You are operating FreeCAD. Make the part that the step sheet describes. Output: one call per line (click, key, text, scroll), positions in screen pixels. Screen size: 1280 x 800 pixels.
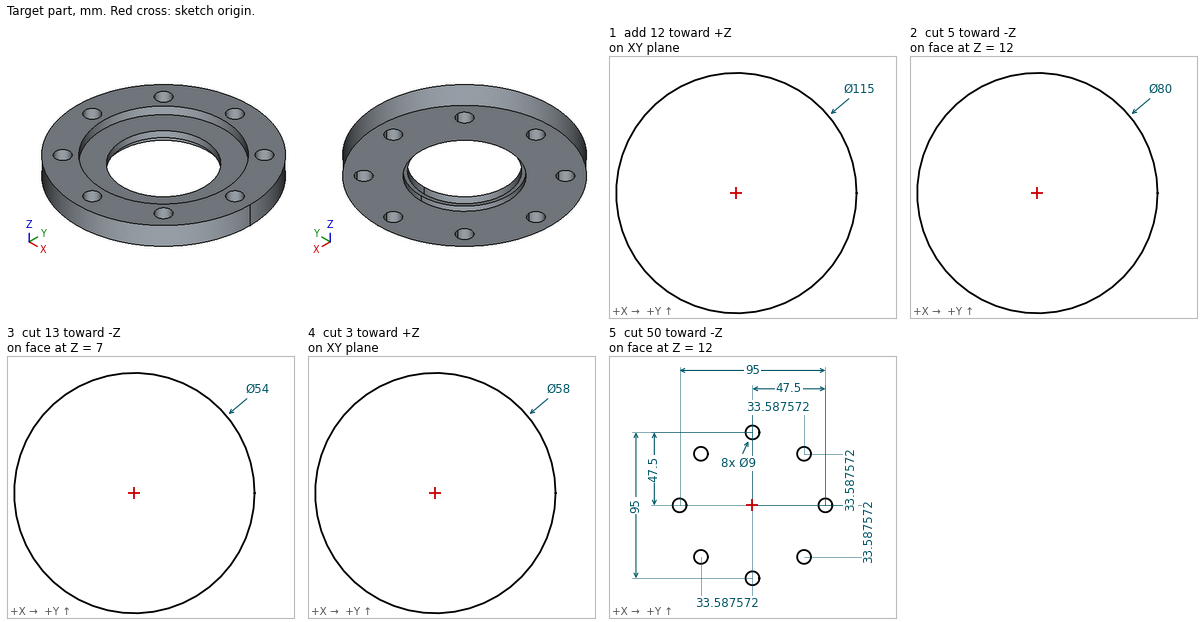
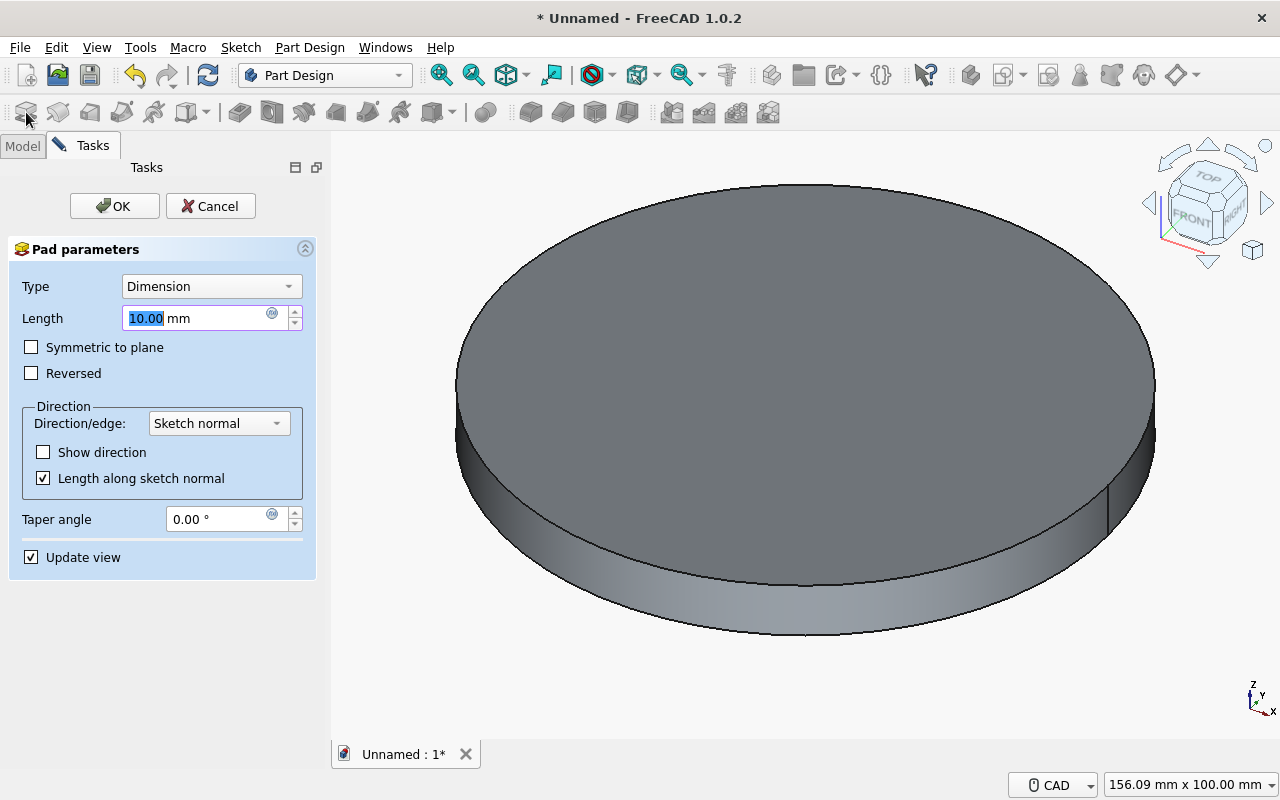
text(12)
key(Tab)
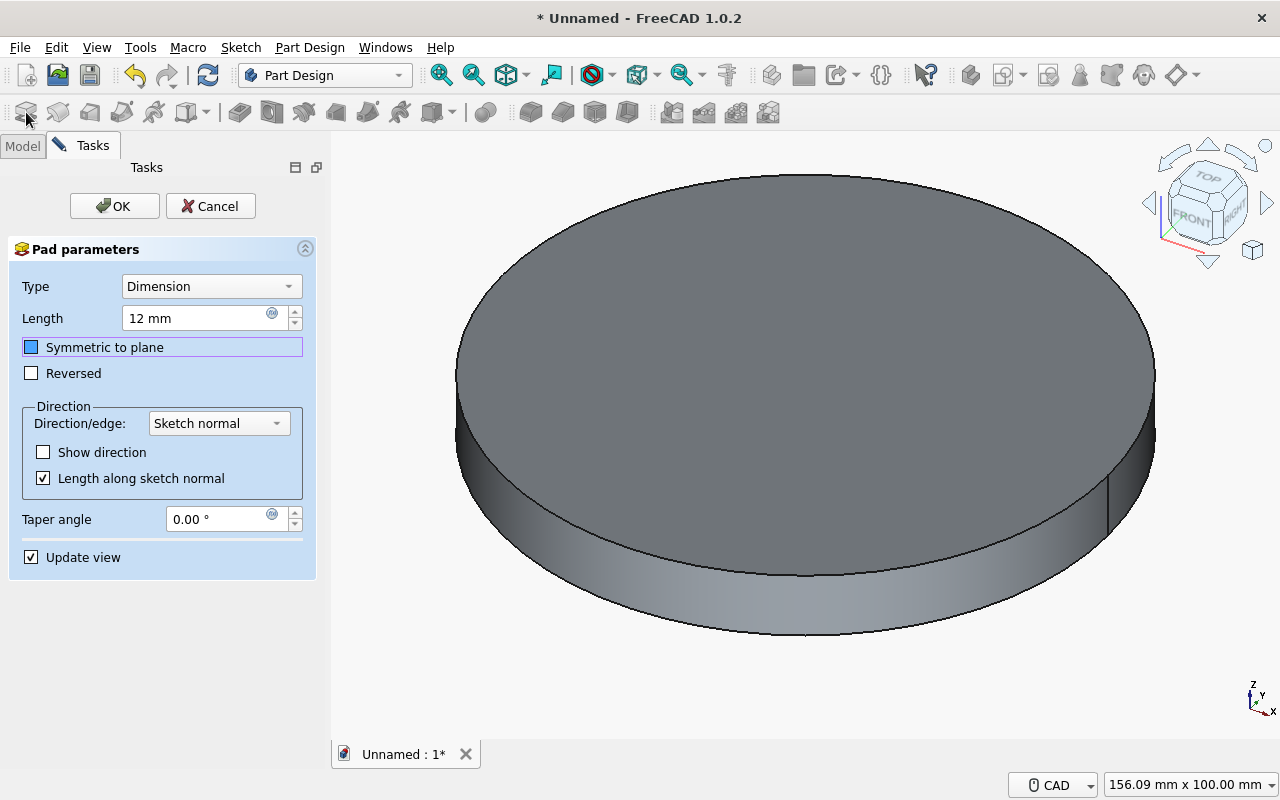
click(115, 206)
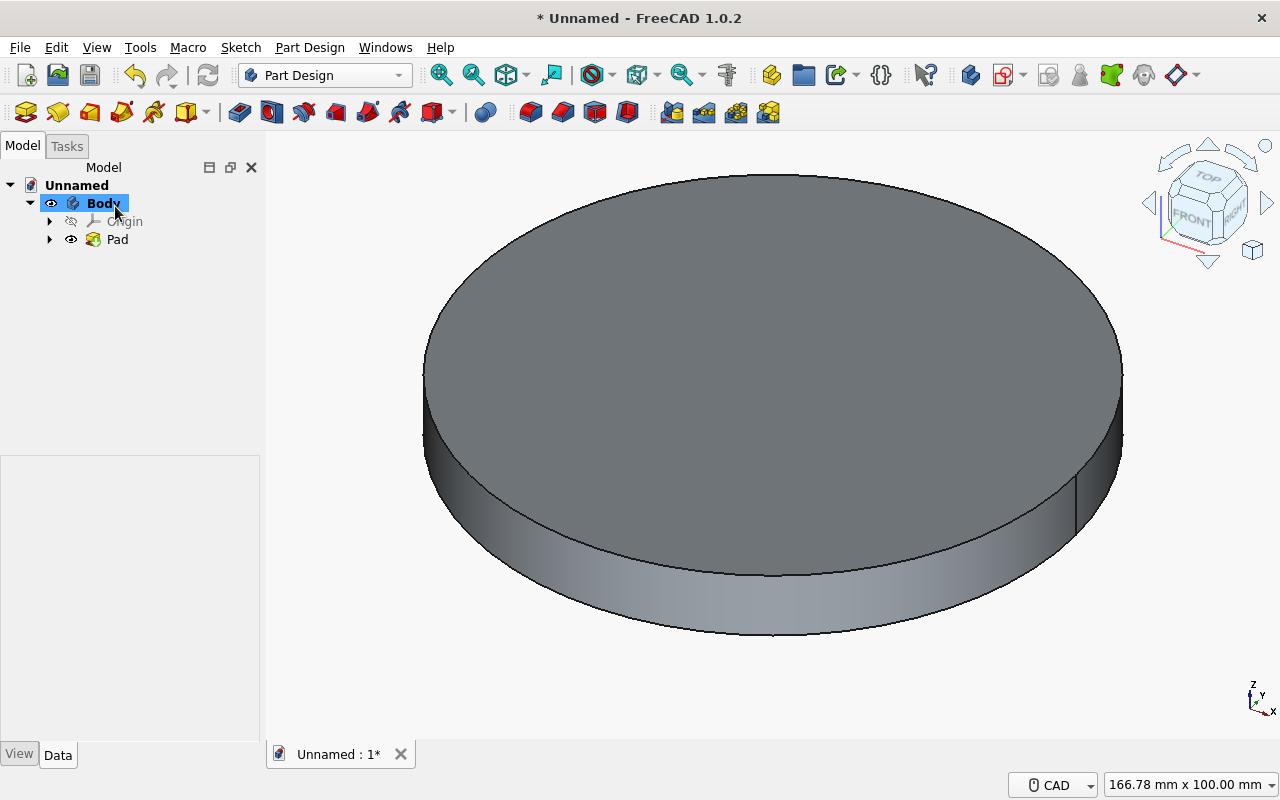
click(442, 76)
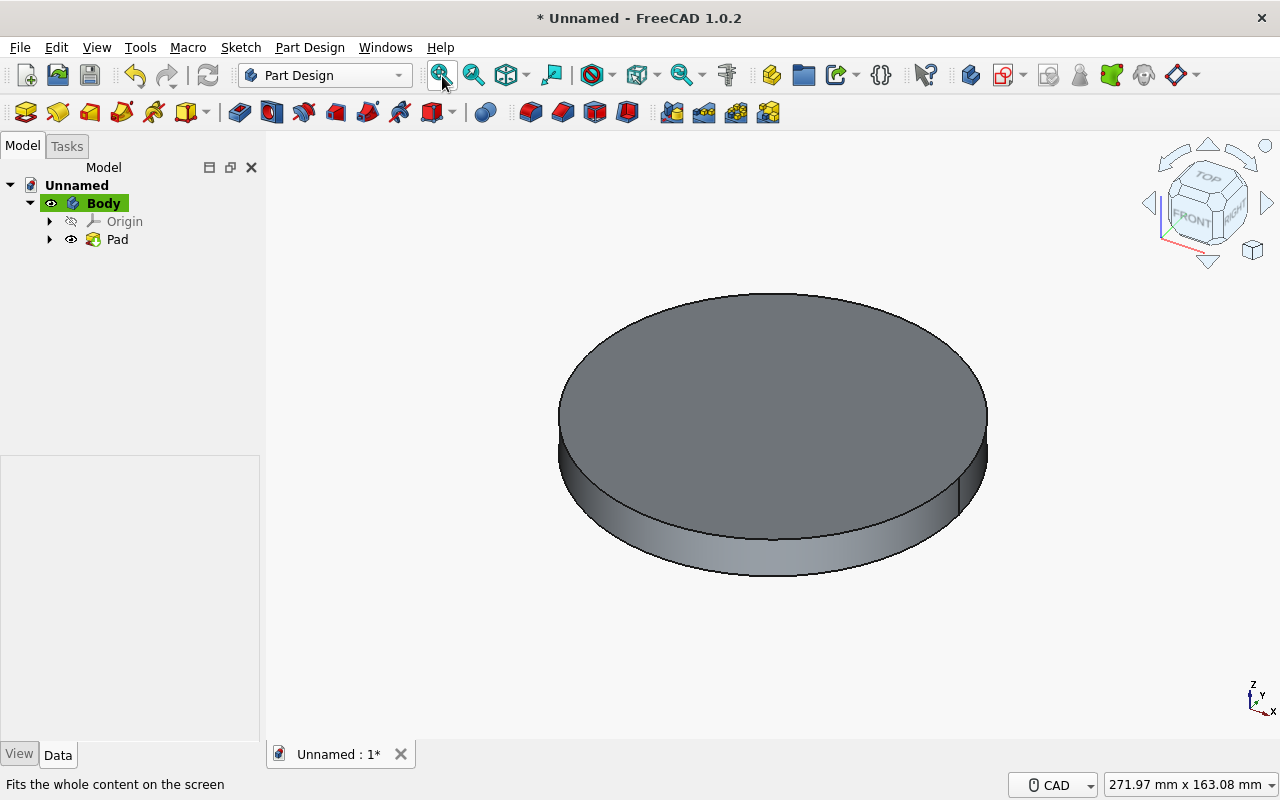
click(773, 416)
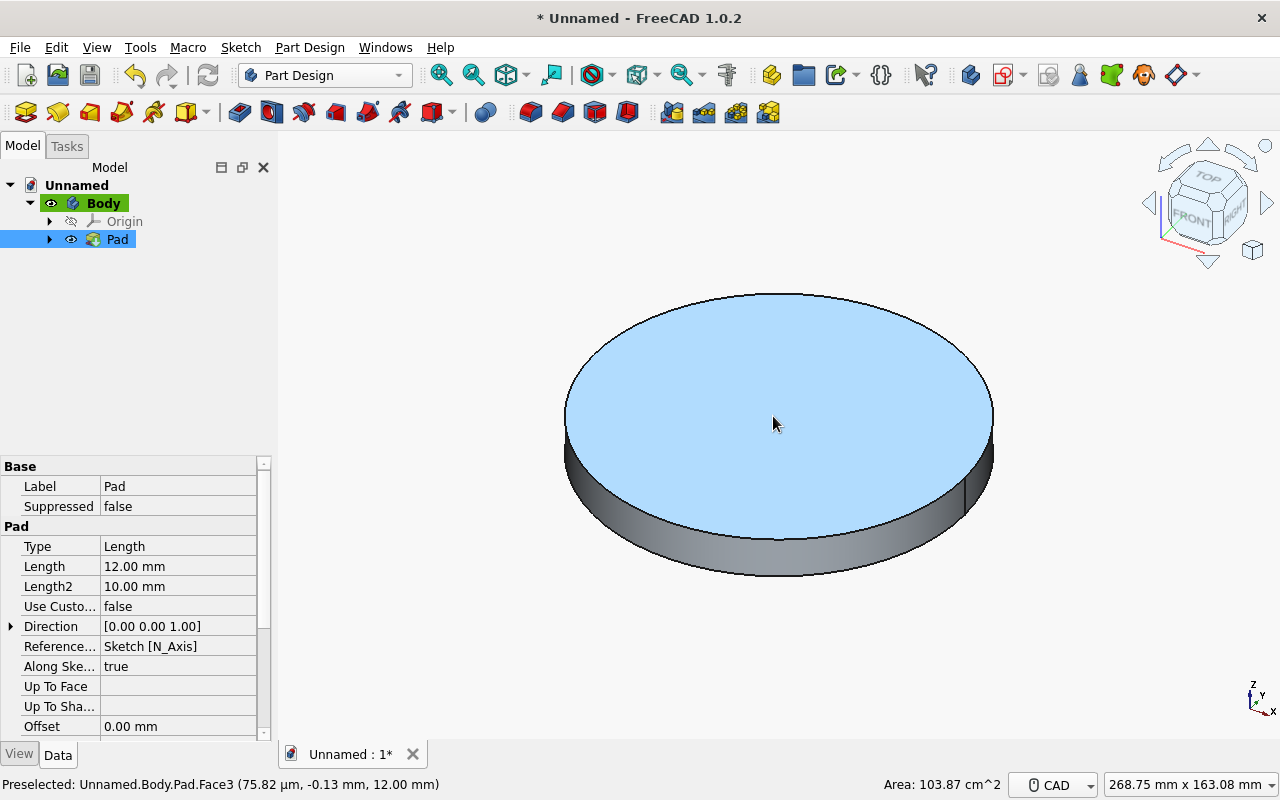
click(1004, 76)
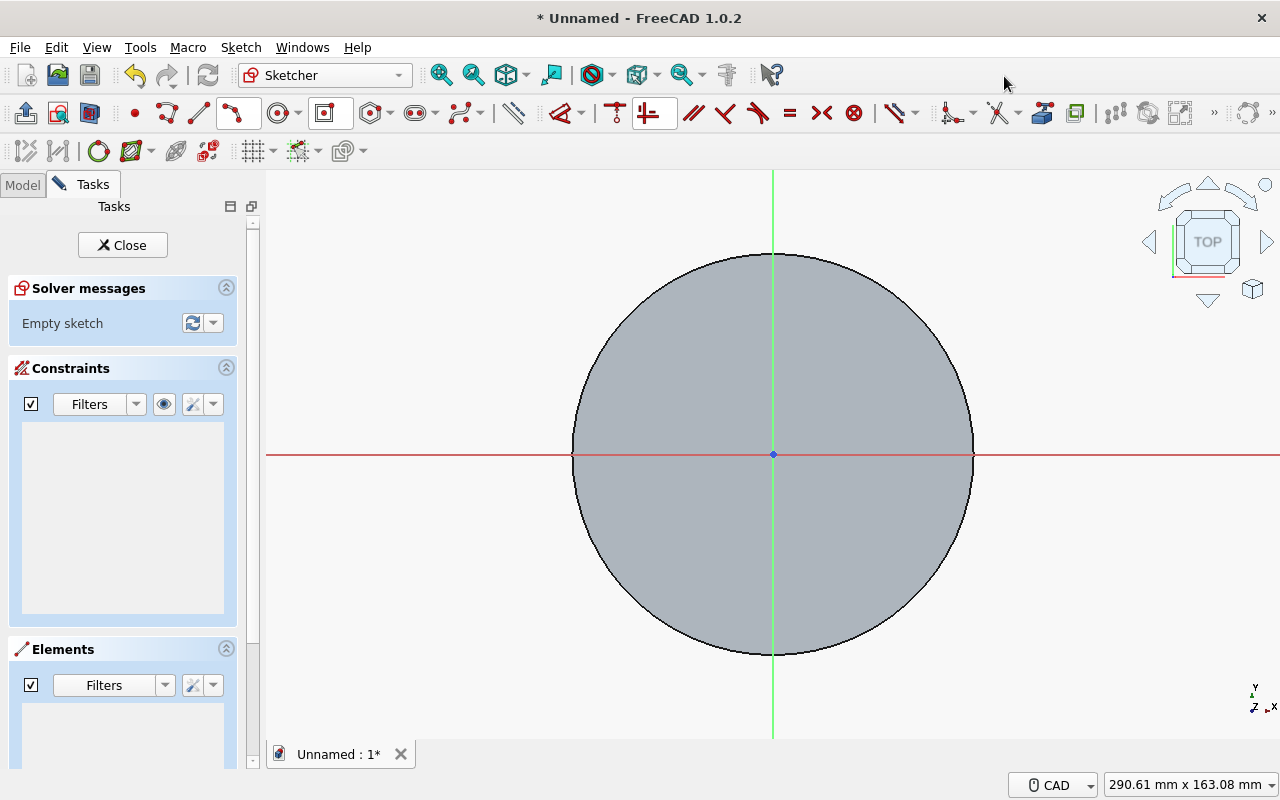
click(278, 114)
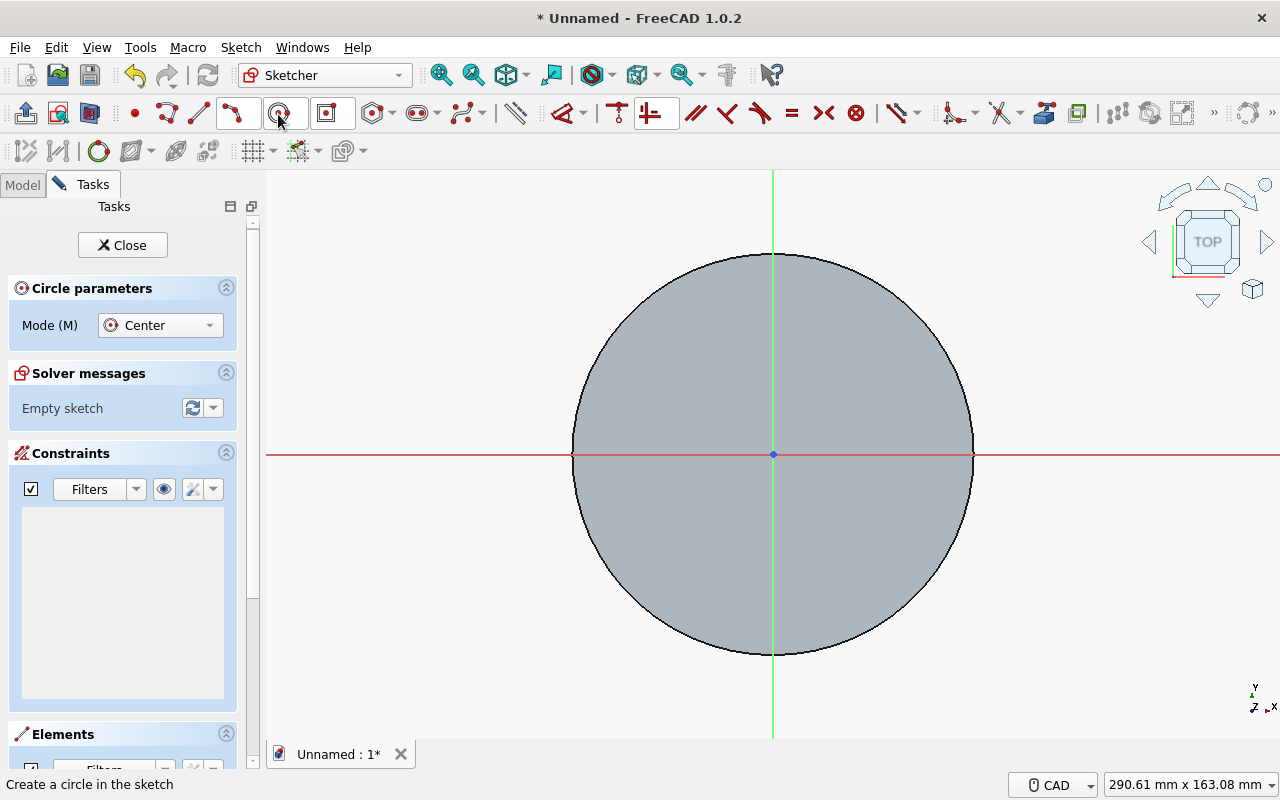
click(773, 454)
move(872, 356)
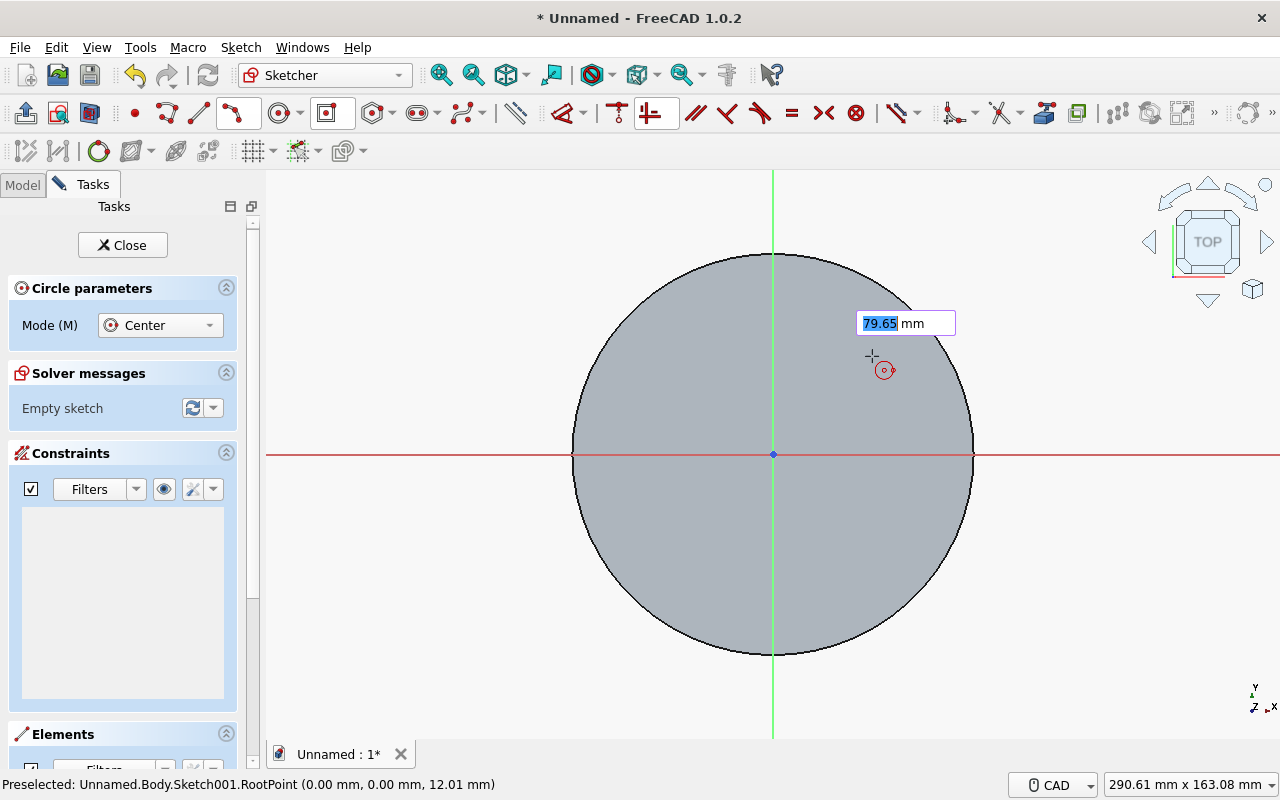
text(80)
key(Return)
key(Escape)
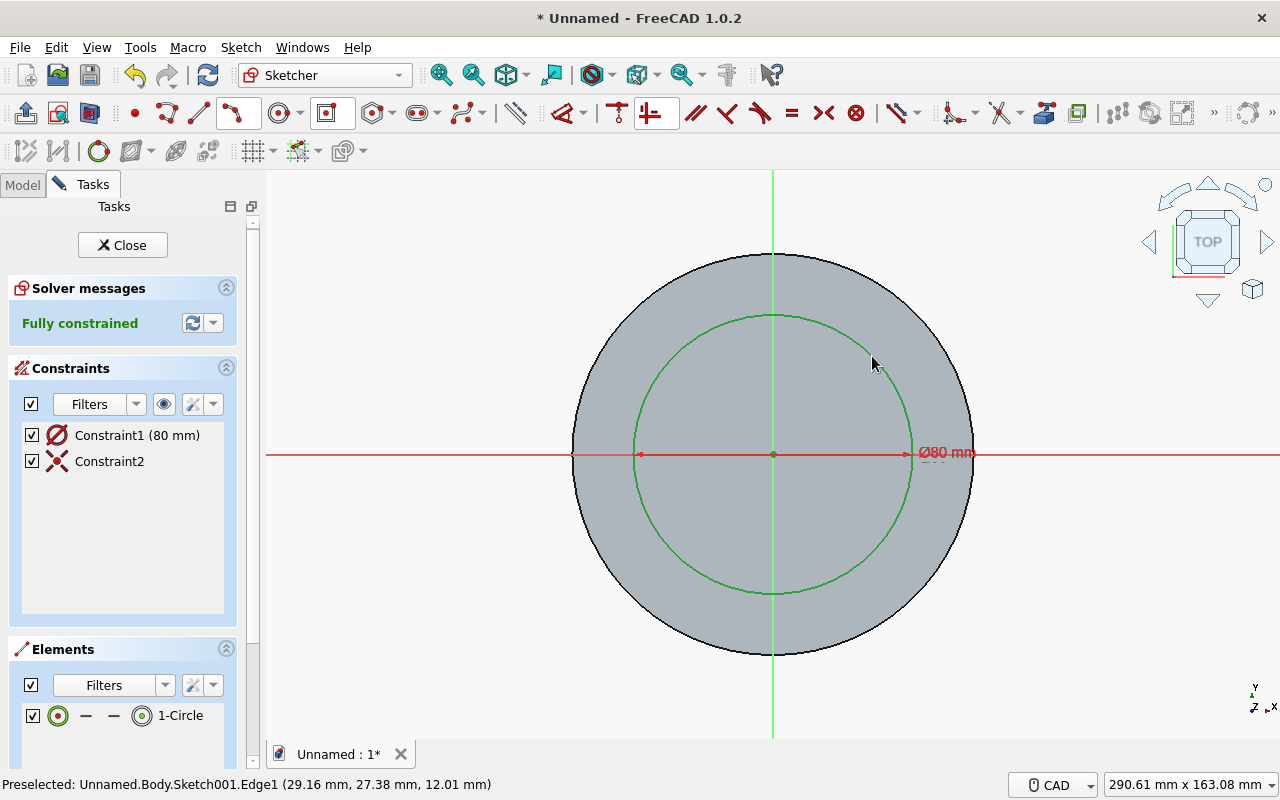
click(123, 245)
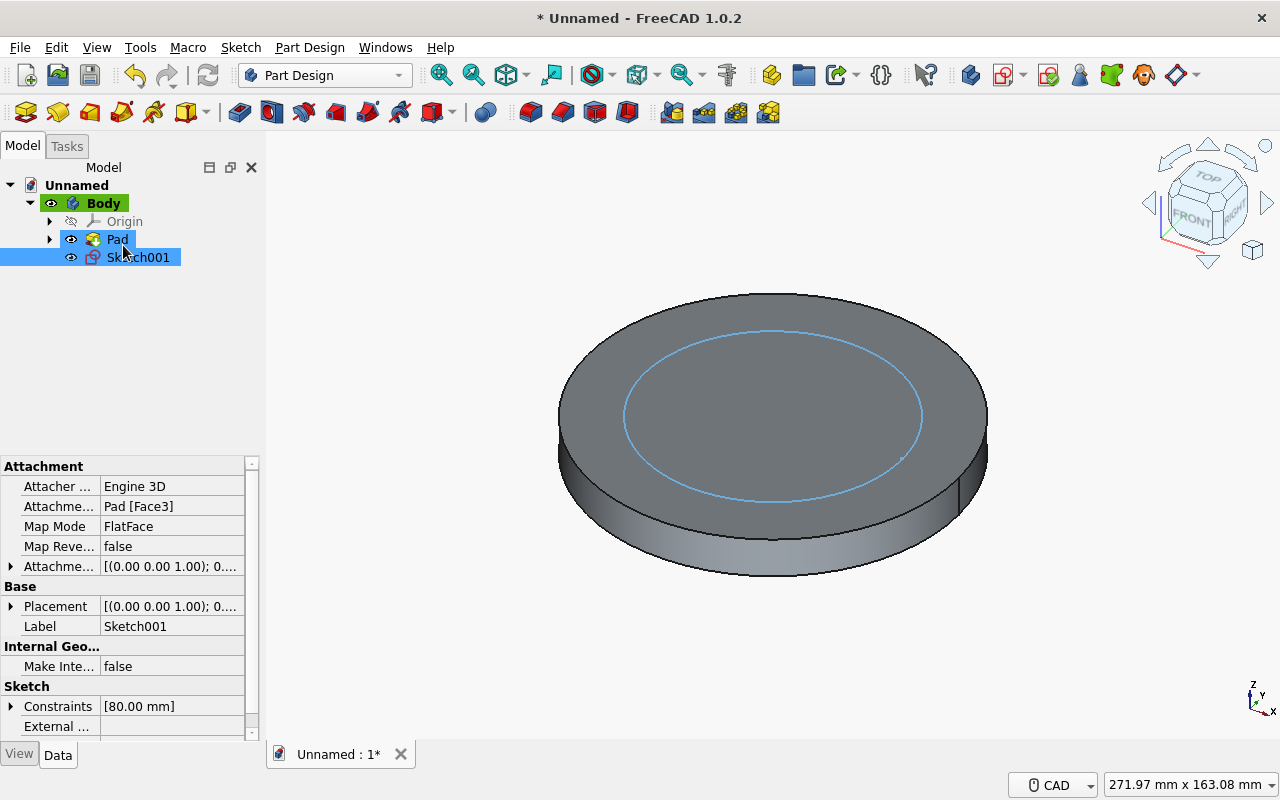
click(240, 112)